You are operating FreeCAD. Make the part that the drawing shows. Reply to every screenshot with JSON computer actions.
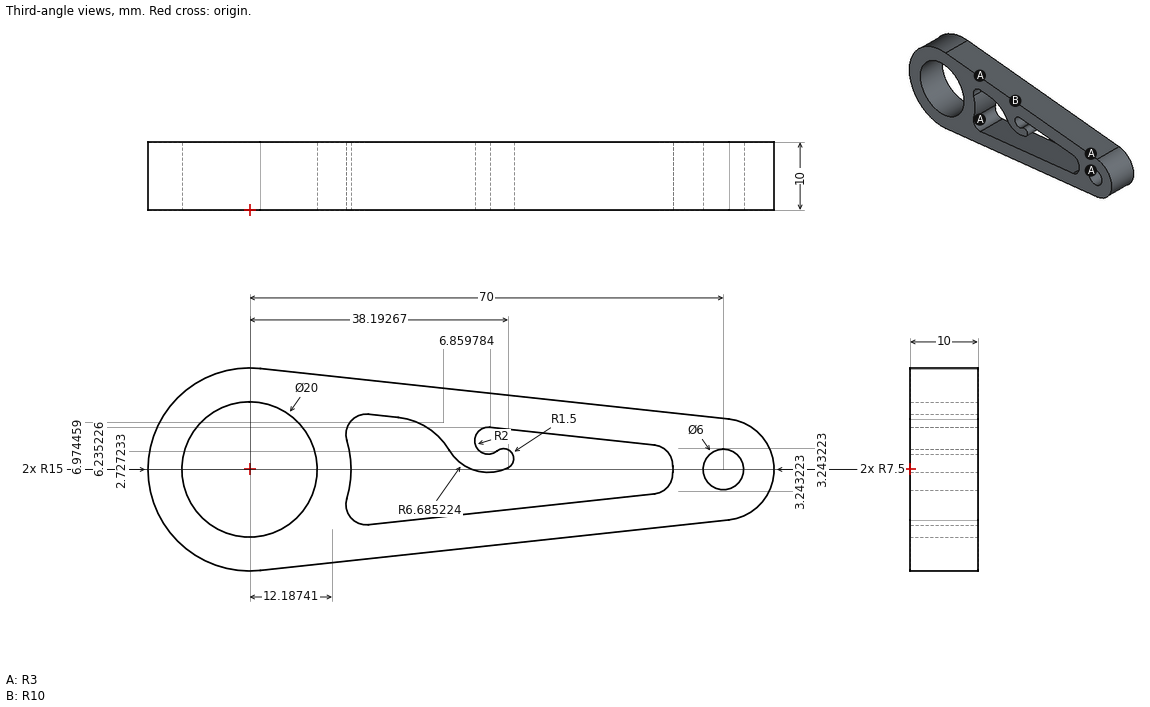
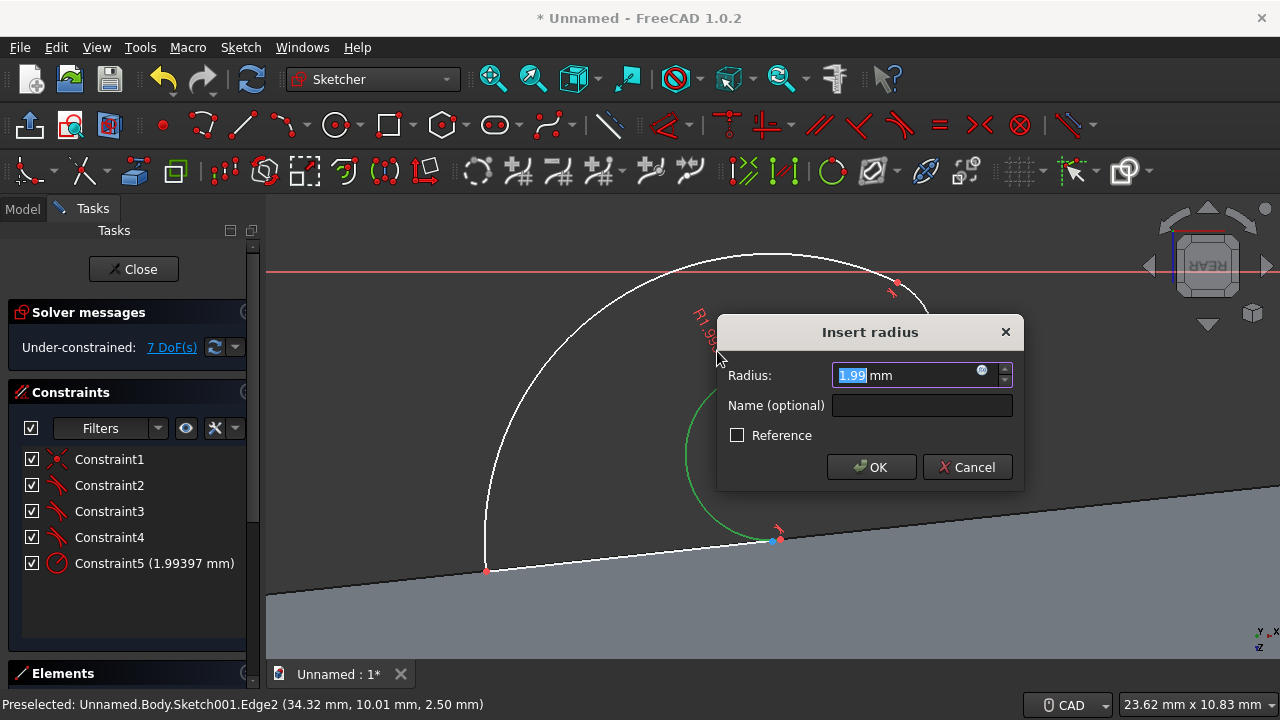
{"action": "type", "text": "2"}
{"action": "key", "text": "Return"}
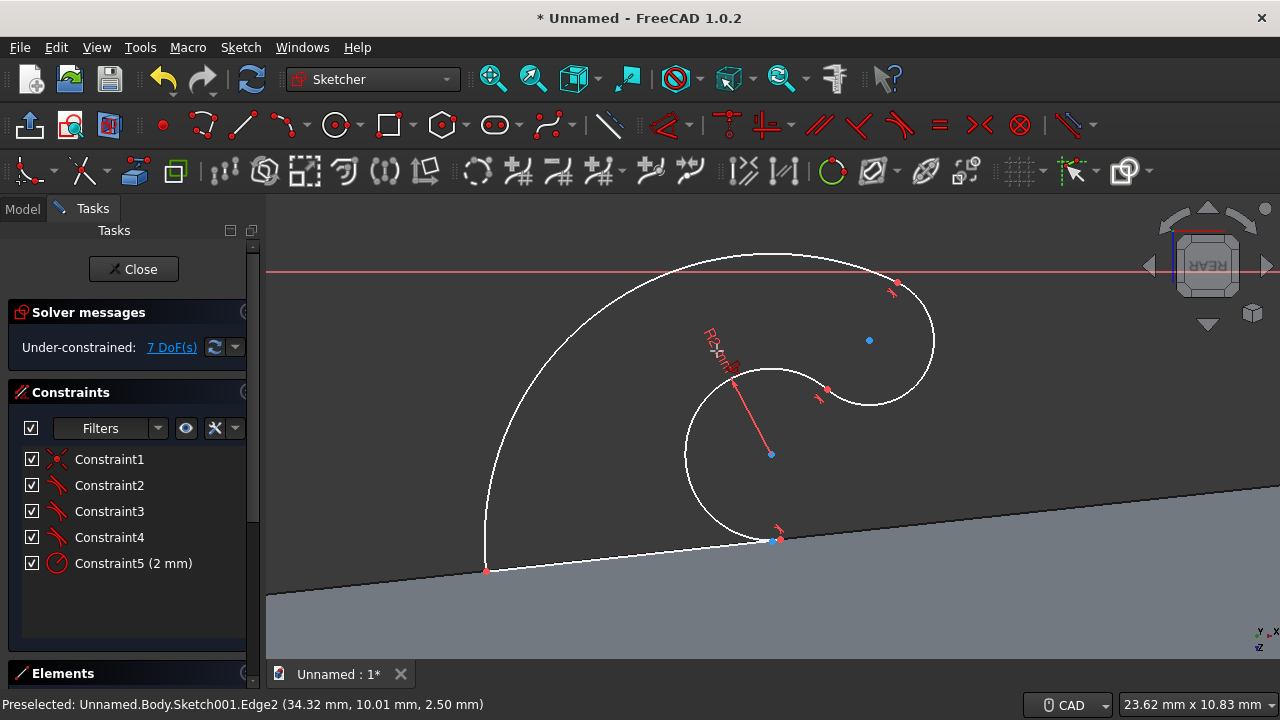
{"action": "left_click", "coordinate": [889, 402]}
{"action": "left_click", "coordinate": [899, 432]}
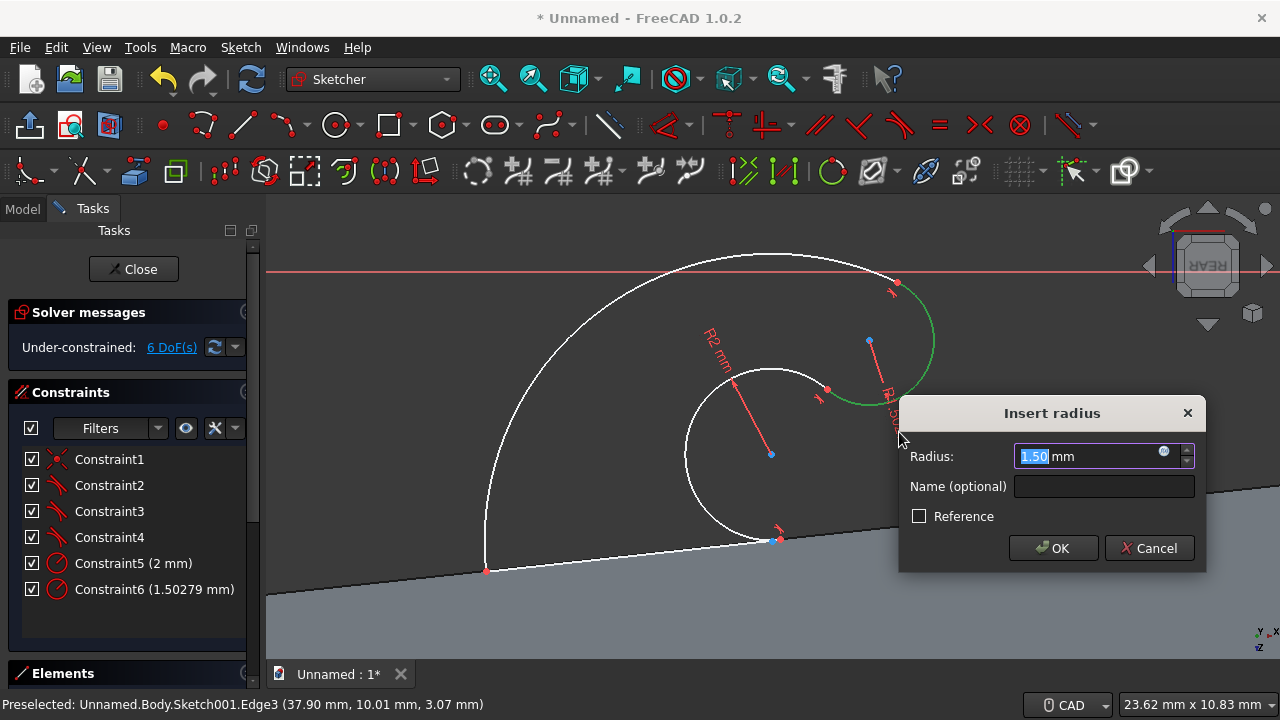
{"action": "type", "text": "1.5"}
{"action": "key", "text": "Return"}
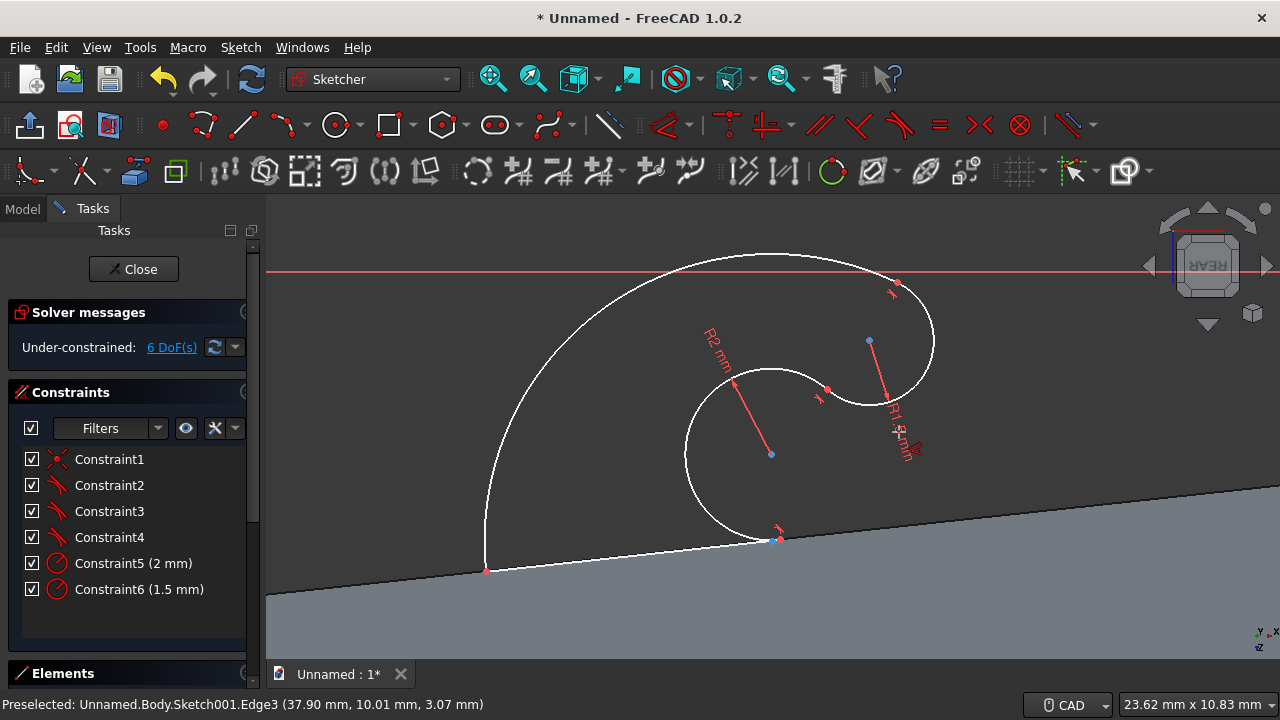
{"action": "left_click", "coordinate": [719, 259]}
{"action": "left_click", "coordinate": [713, 228]}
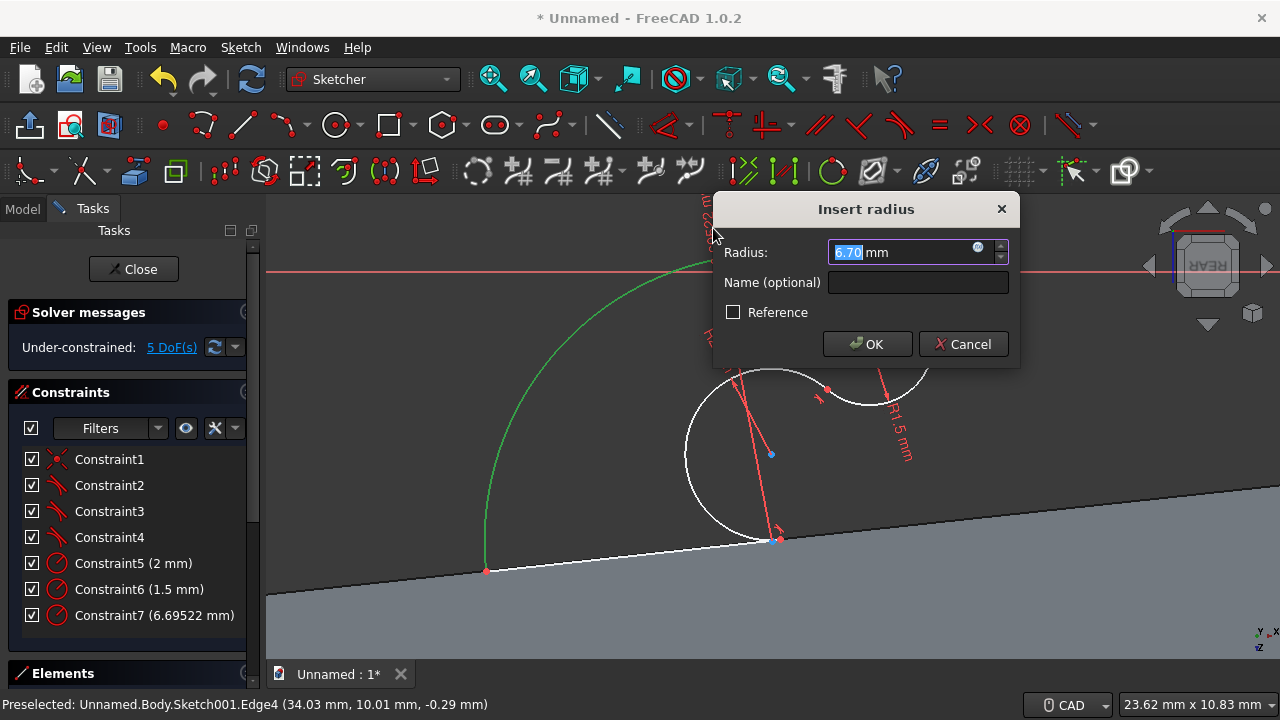
{"action": "type", "text": "6.685224"}
{"action": "key", "text": "Return"}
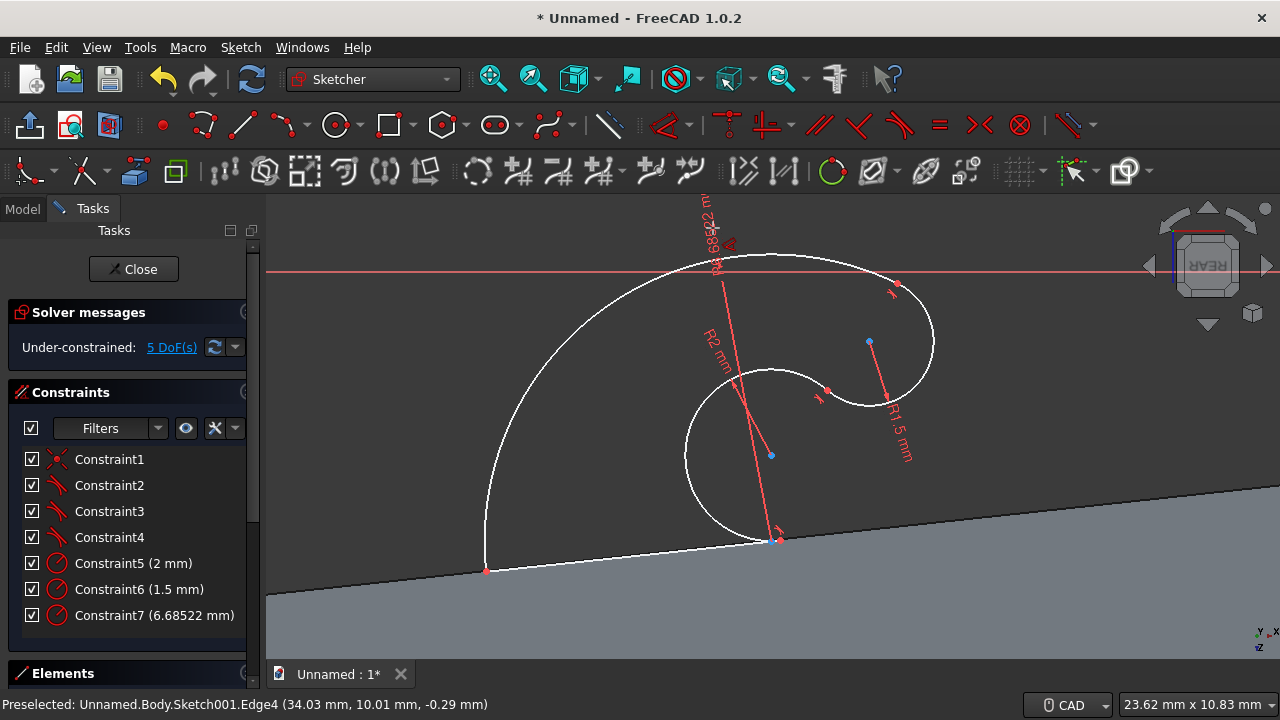
{"action": "left_click", "coordinate": [486, 572]}
{"action": "left_click", "coordinate": [520, 353]}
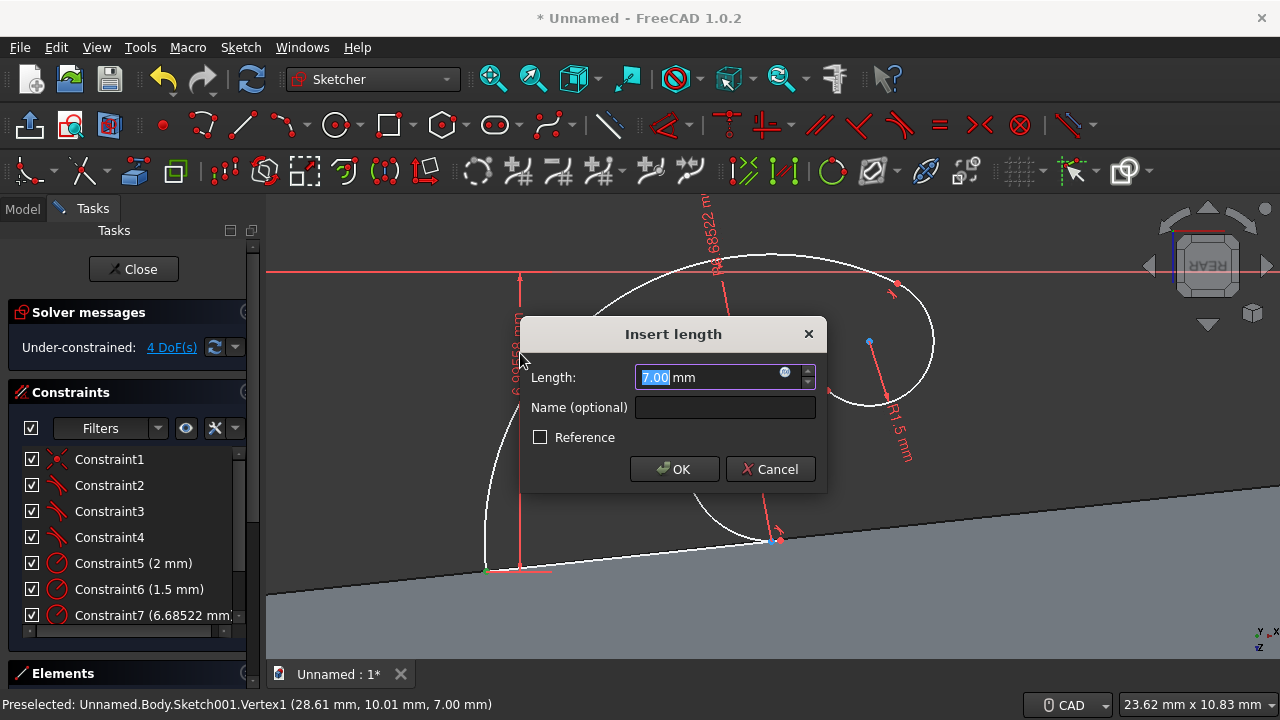
{"action": "type", "text": "6.974459"}
{"action": "key", "text": "Return"}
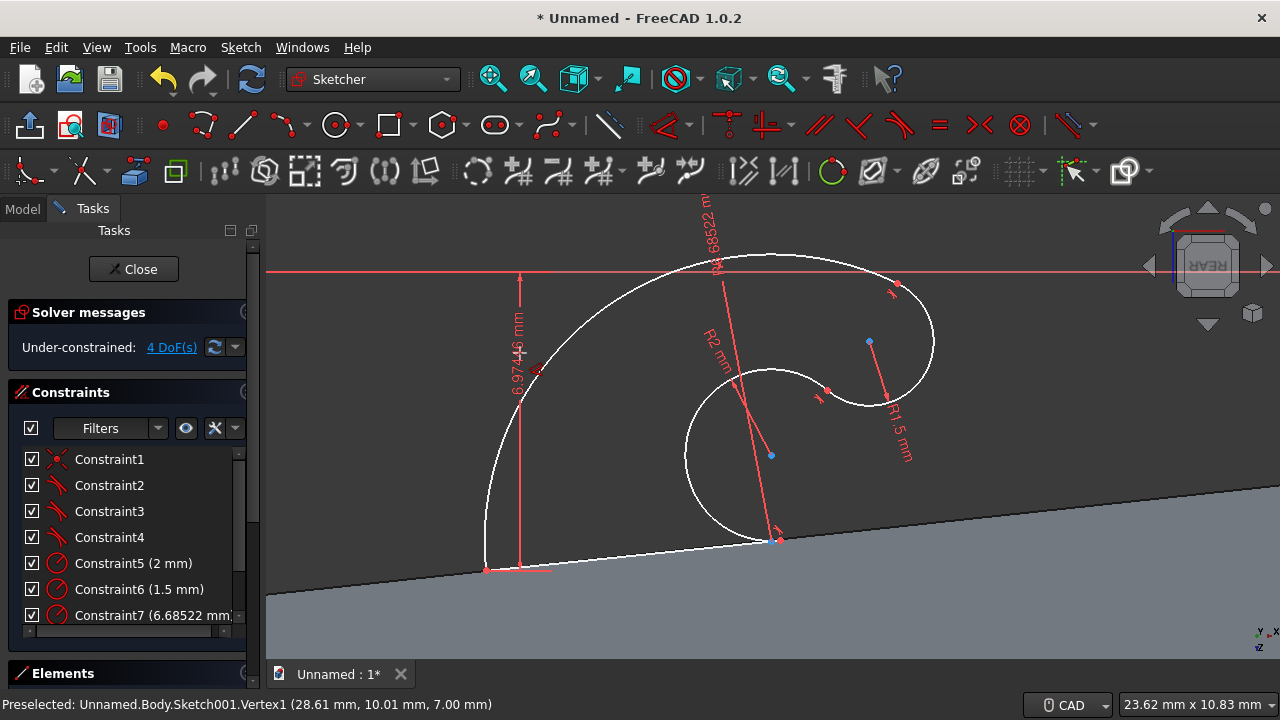
{"action": "scroll", "coordinate": [780, 541], "scroll_direction": "up", "scroll_amount": 2}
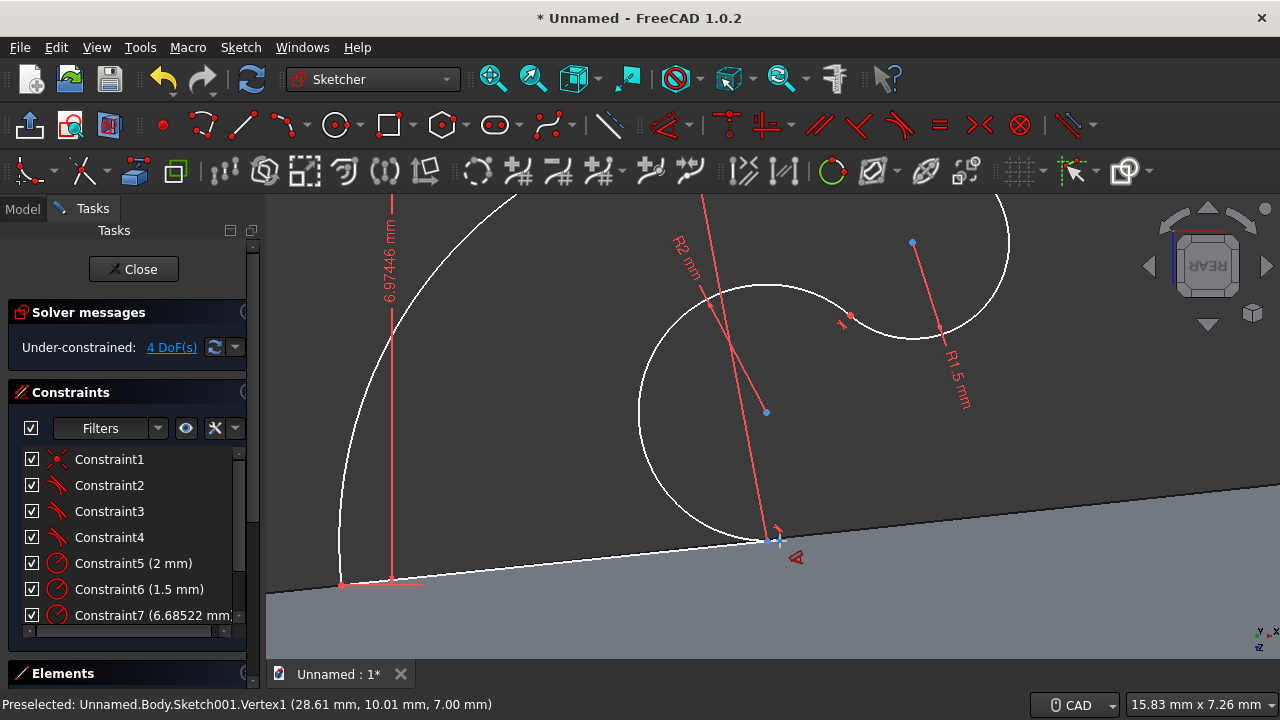
{"action": "left_click", "coordinate": [780, 540]}
{"action": "left_click", "coordinate": [814, 381]}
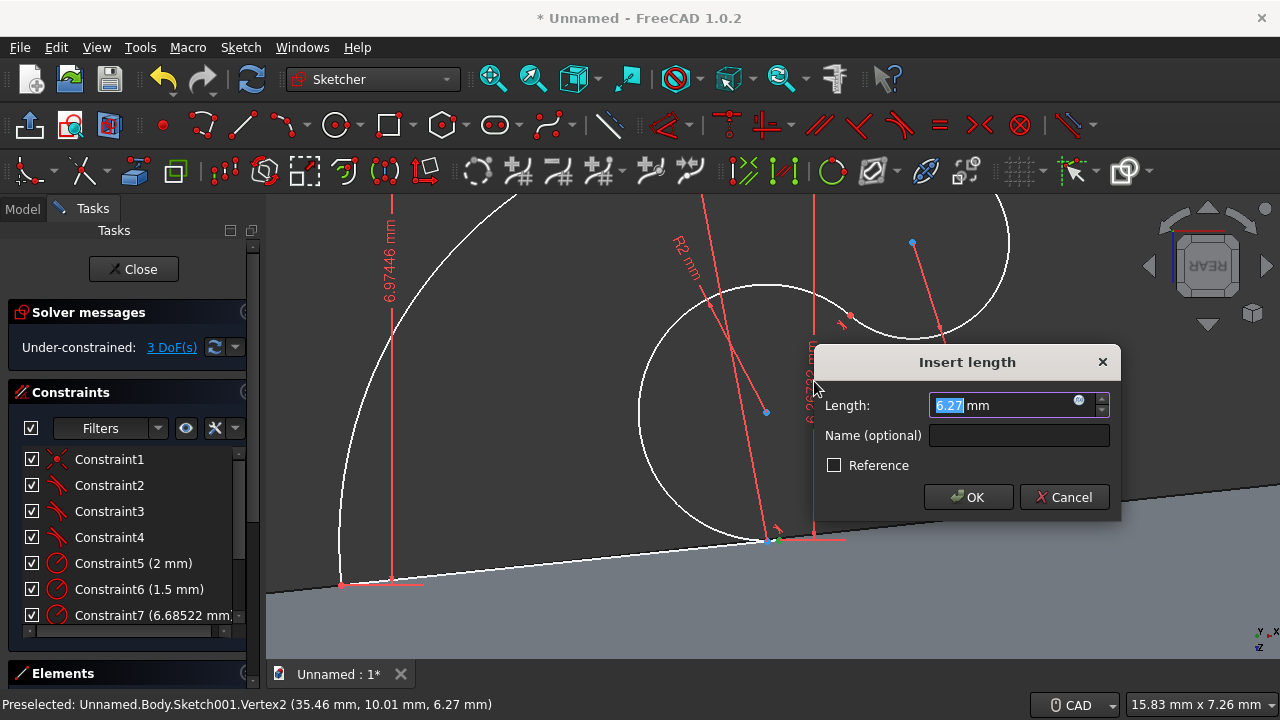
{"action": "type", "text": "6.235226"}
{"action": "key", "text": "Return"}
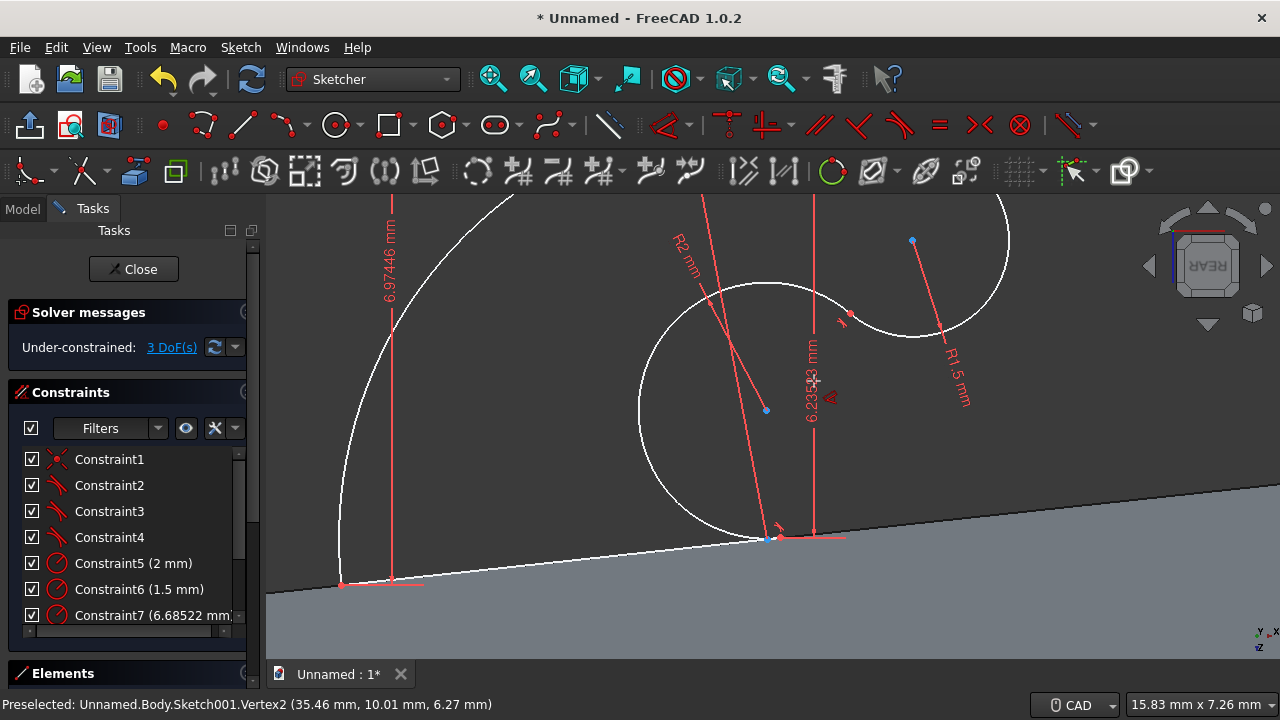
{"action": "left_click", "coordinate": [850, 314]}
{"action": "left_click", "coordinate": [884, 268]}